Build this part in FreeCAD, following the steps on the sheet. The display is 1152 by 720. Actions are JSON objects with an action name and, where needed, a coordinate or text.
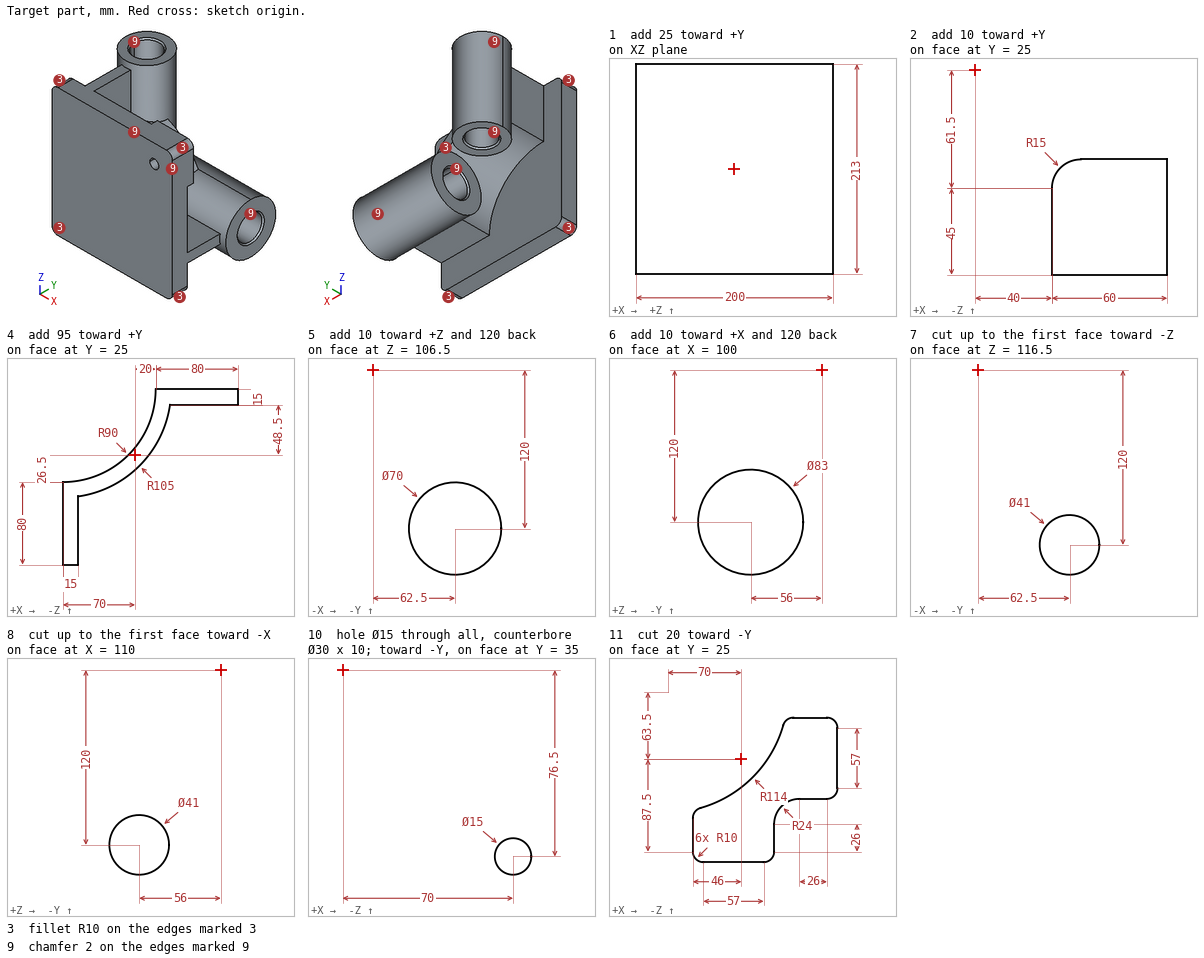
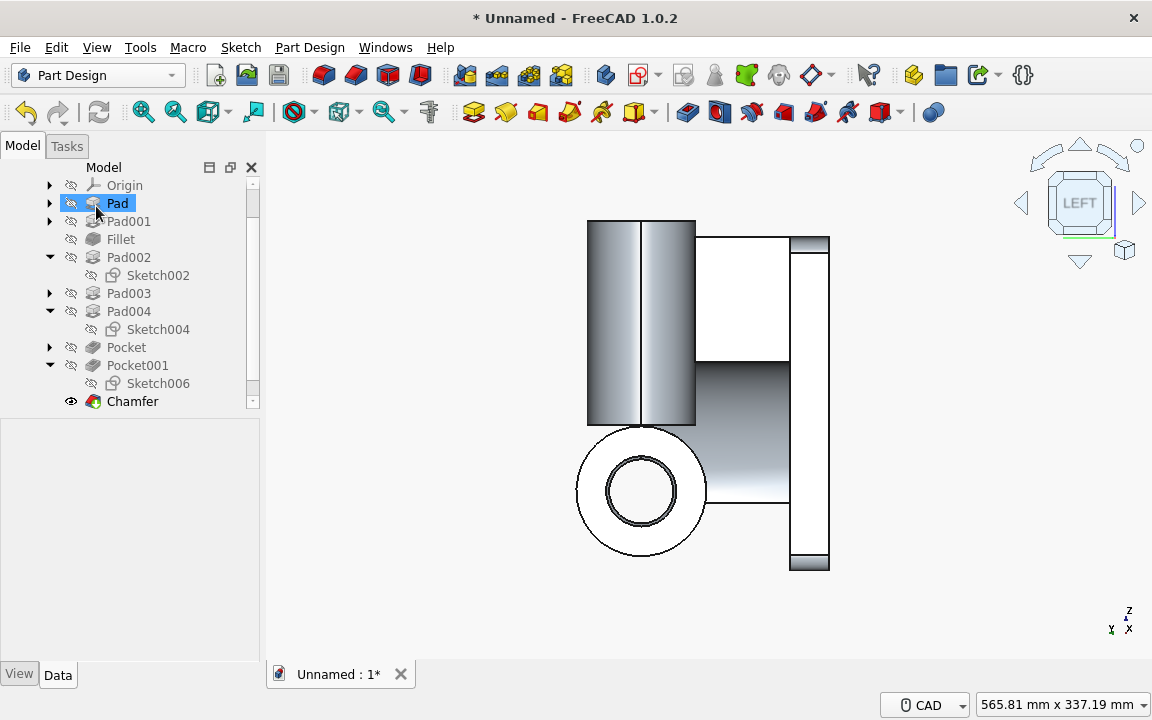
{"action": "key", "text": "4"}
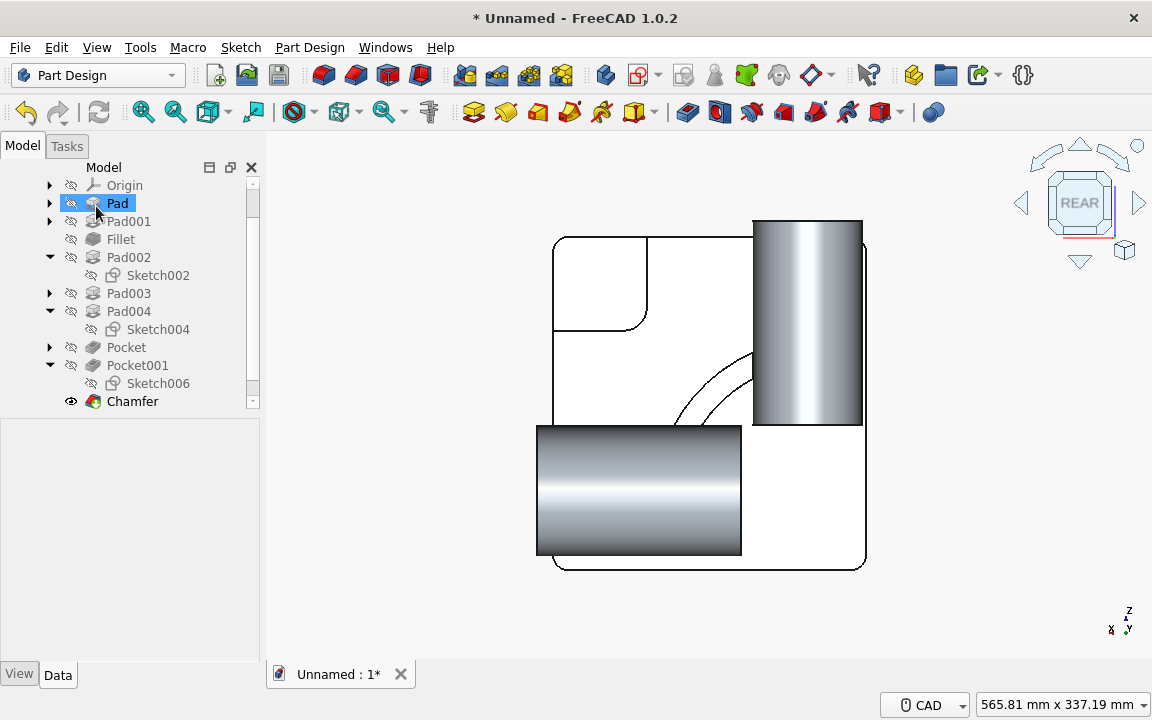
{"action": "left_click", "coordinate": [600, 283]}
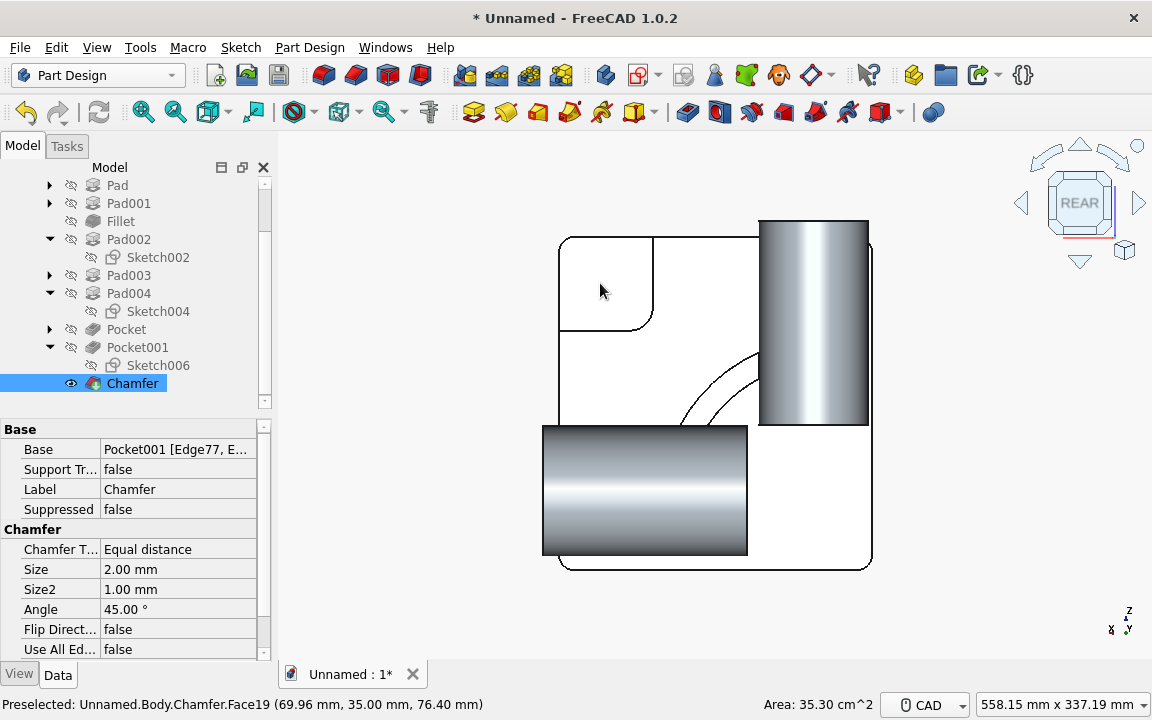
{"action": "left_click", "coordinate": [638, 76]}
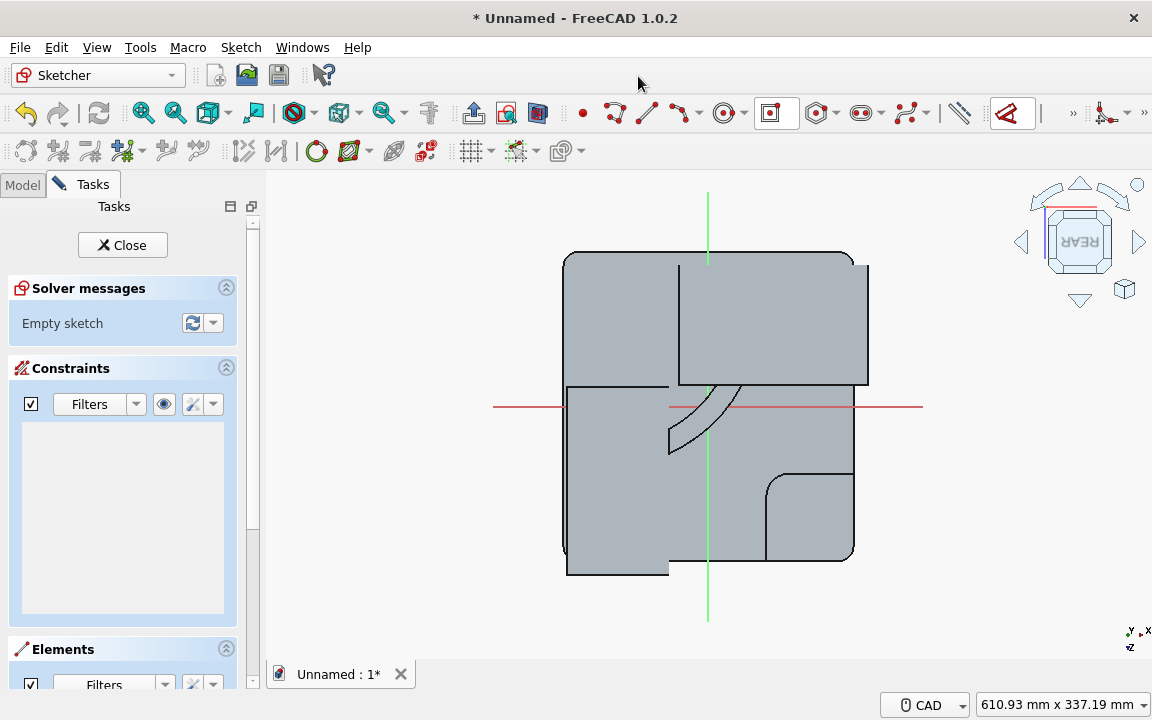
{"action": "left_click", "coordinate": [538, 114]}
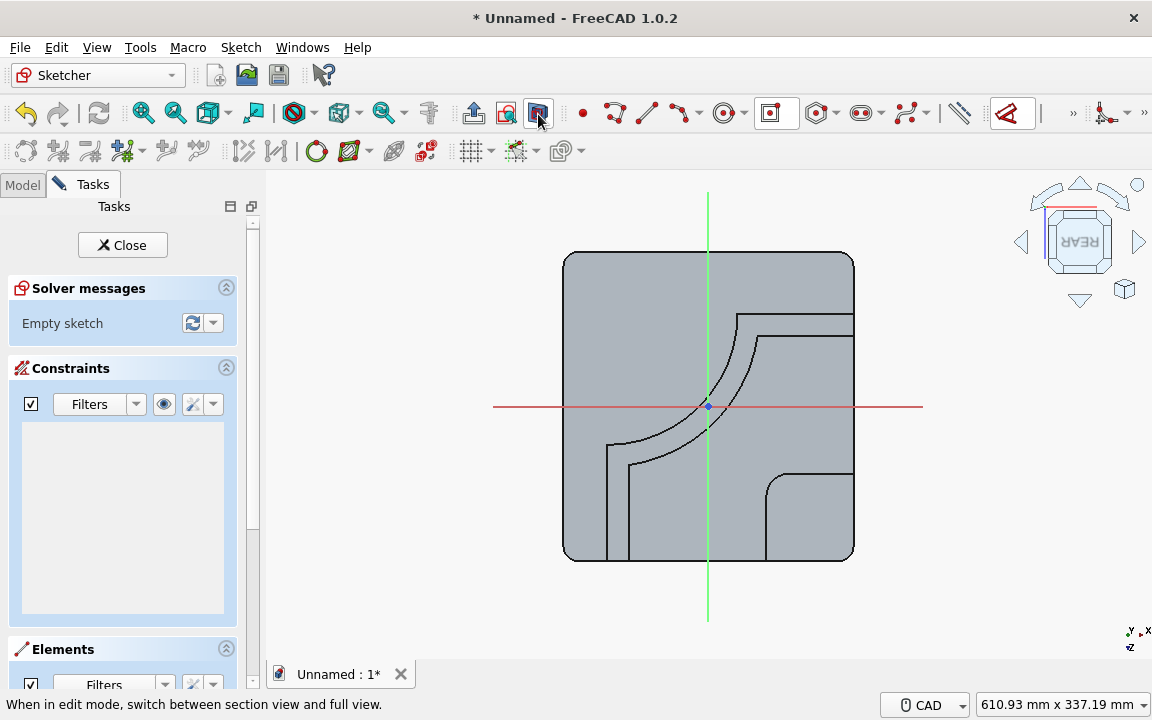
{"action": "scroll", "coordinate": [824, 526], "scroll_direction": "up", "scroll_amount": 13}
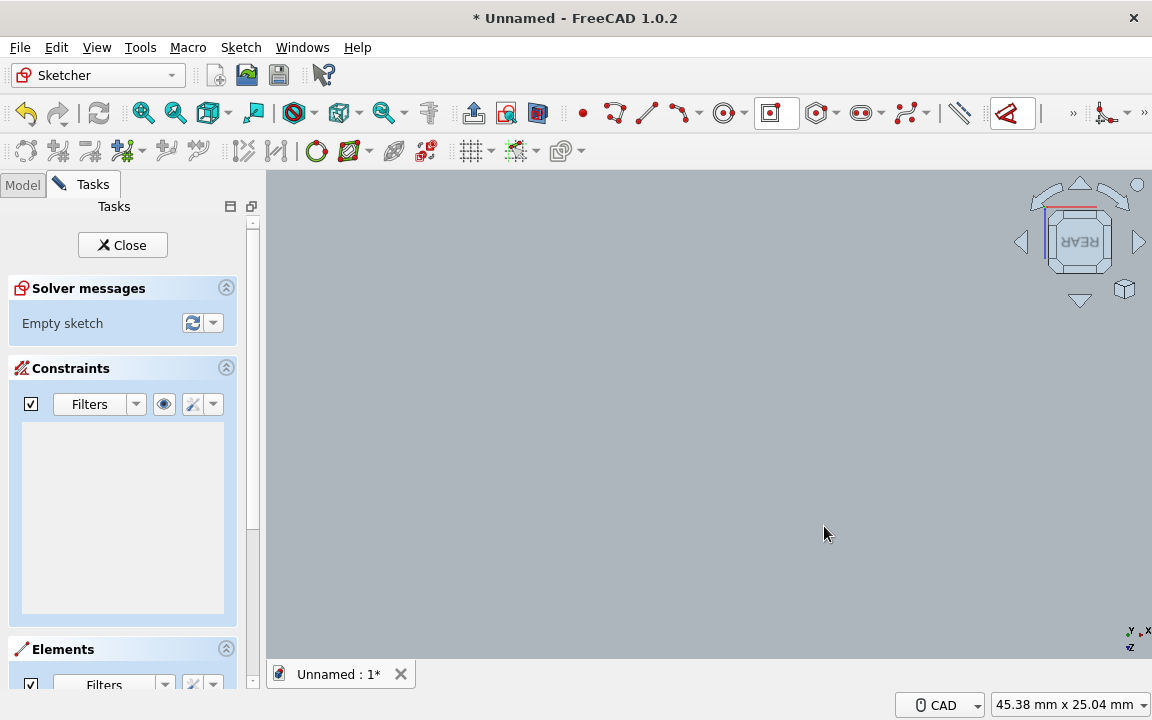
{"action": "left_click", "coordinate": [724, 114]}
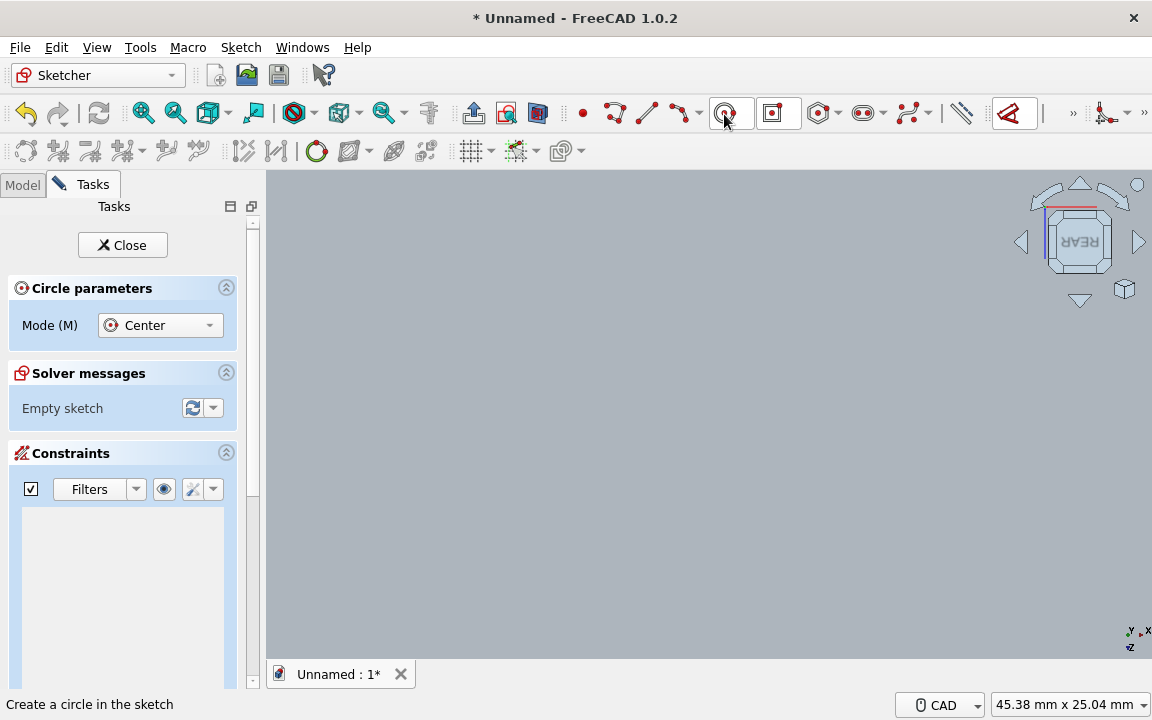
{"action": "left_click", "coordinate": [628, 402]}
{"action": "mouse_move", "coordinate": [731, 298]}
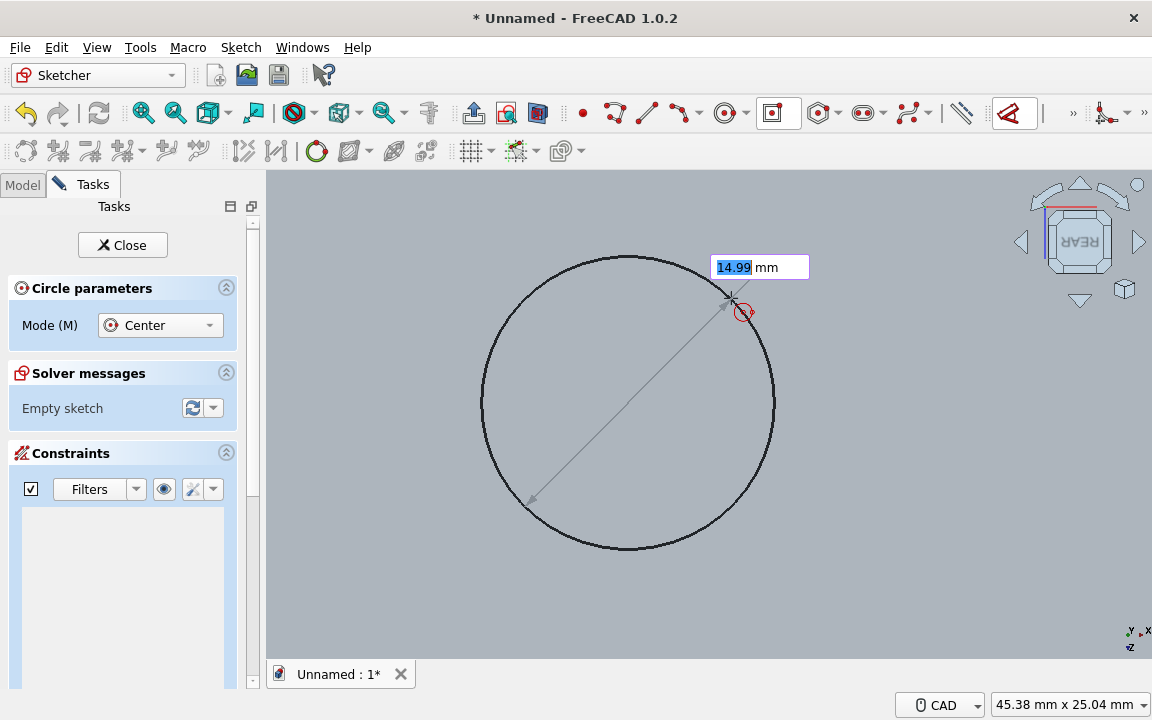
{"action": "type", "text": "15"}
{"action": "key", "text": "Return"}
{"action": "key", "text": "Escape"}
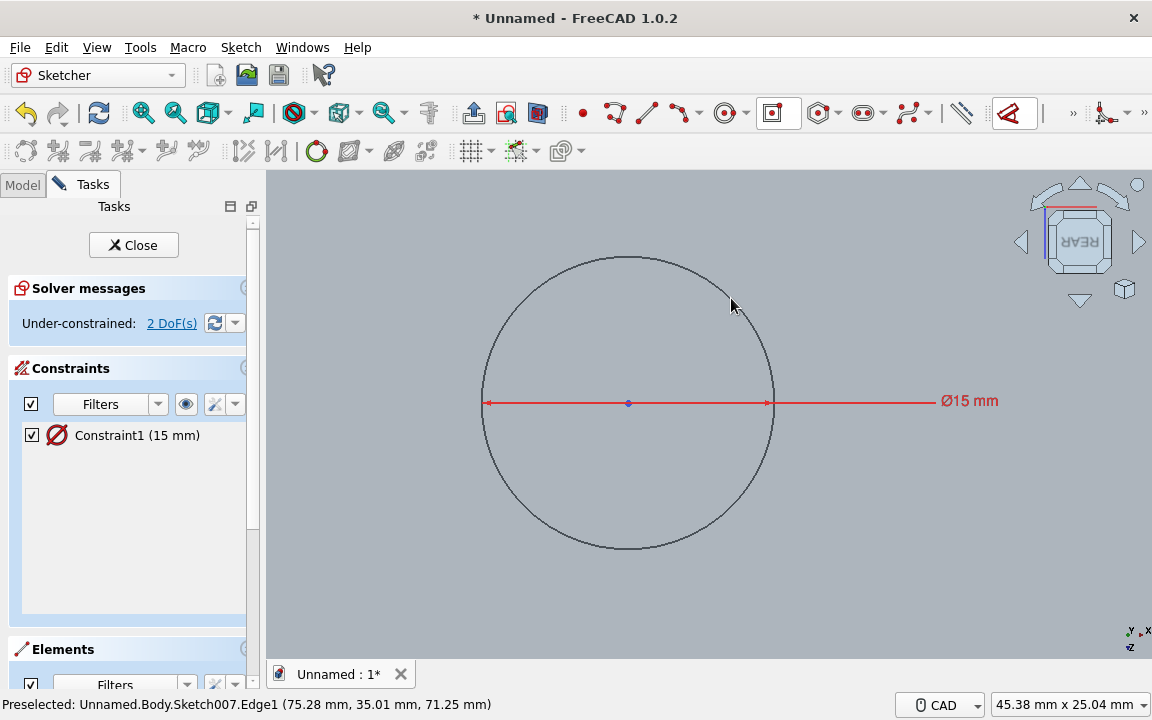
{"action": "left_click", "coordinate": [628, 403]}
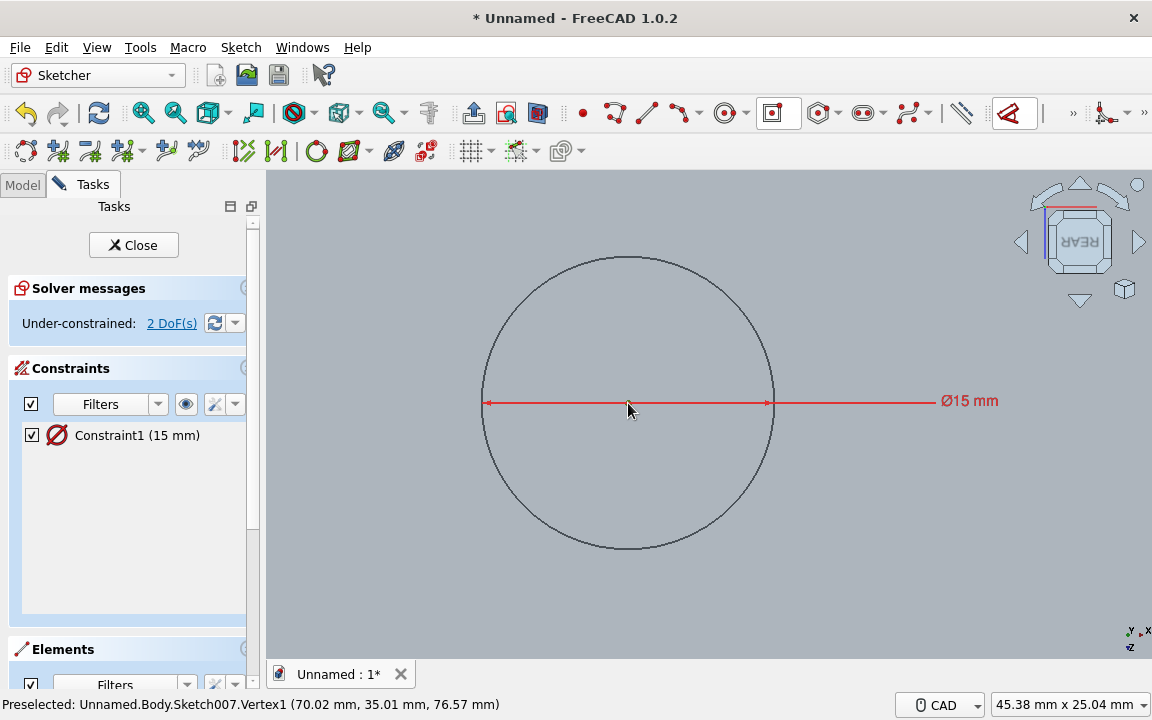
{"action": "key", "text": "l"}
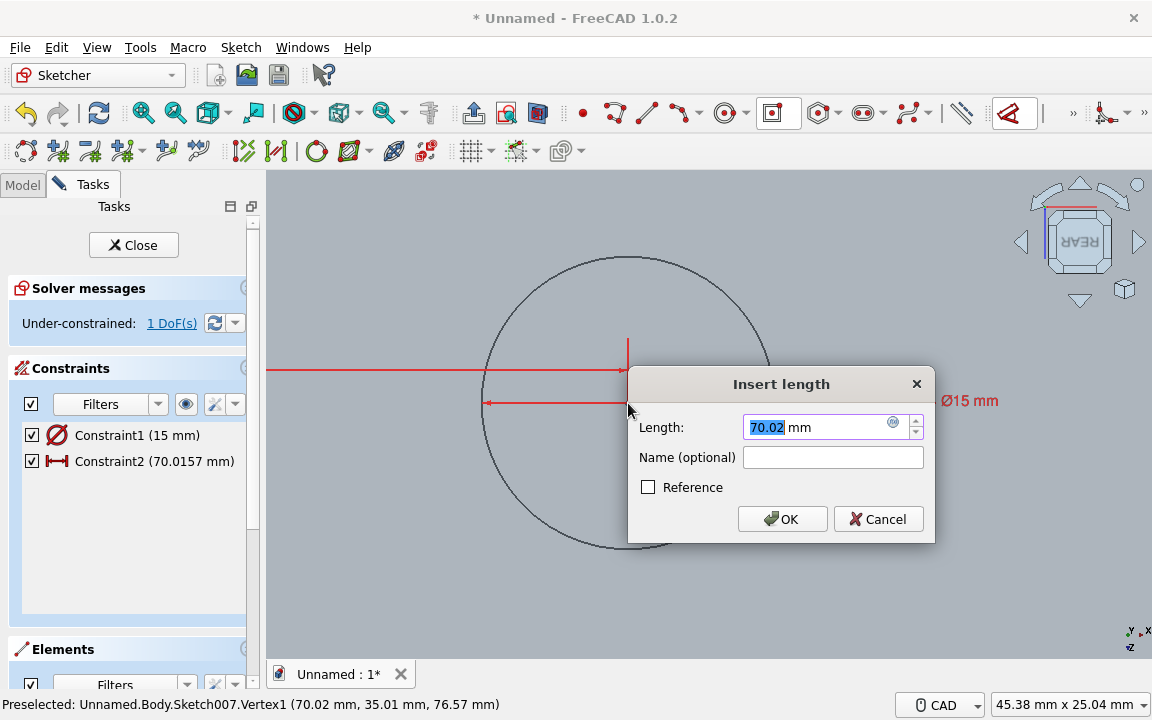
{"action": "type", "text": "70"}
{"action": "key", "text": "Return"}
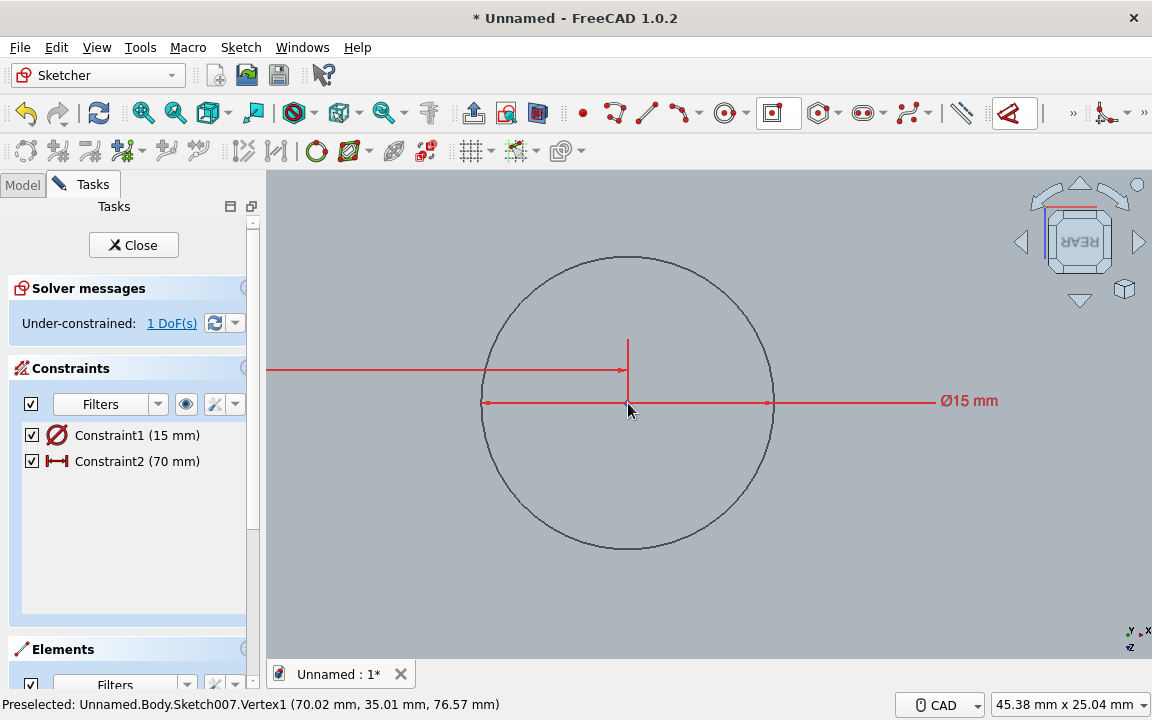
{"action": "left_click", "coordinate": [628, 403]}